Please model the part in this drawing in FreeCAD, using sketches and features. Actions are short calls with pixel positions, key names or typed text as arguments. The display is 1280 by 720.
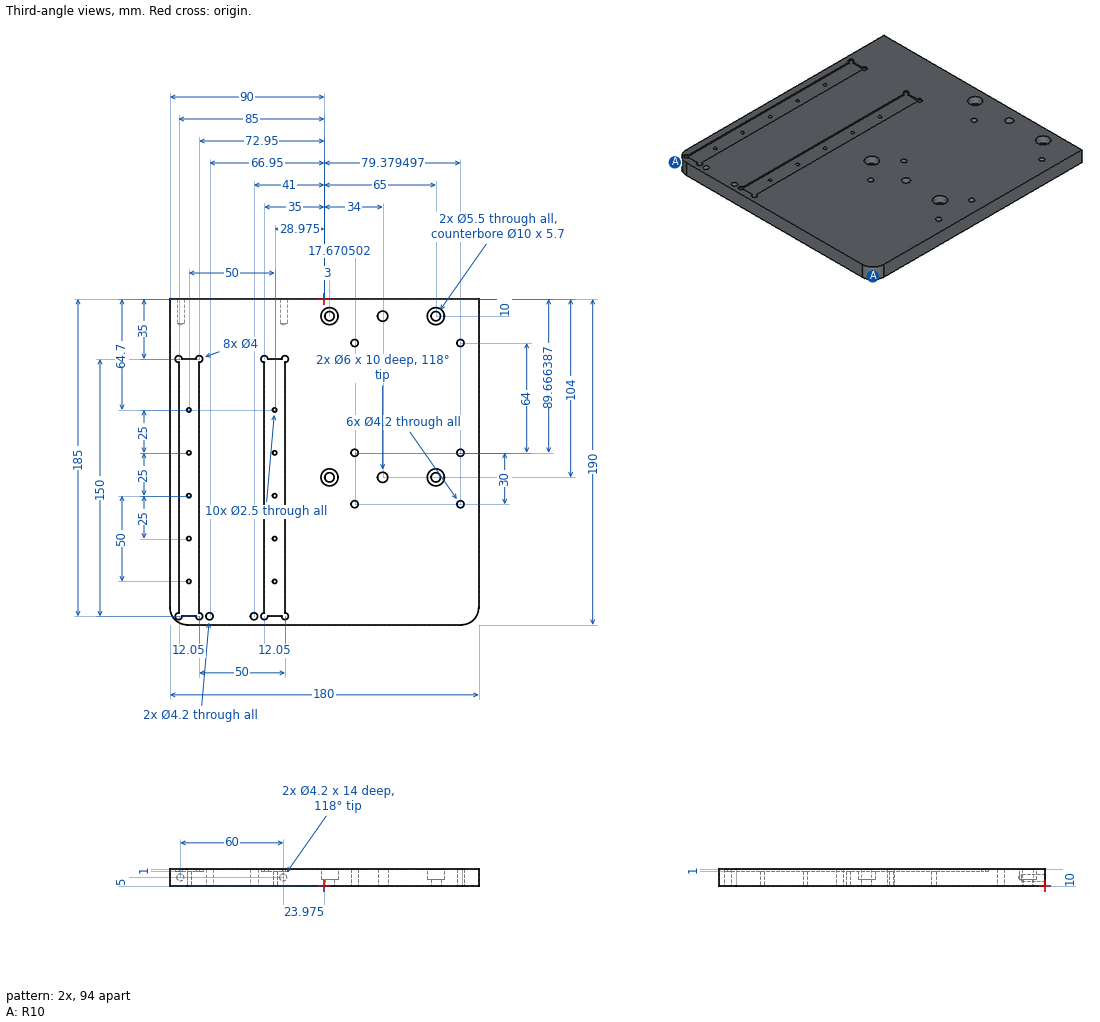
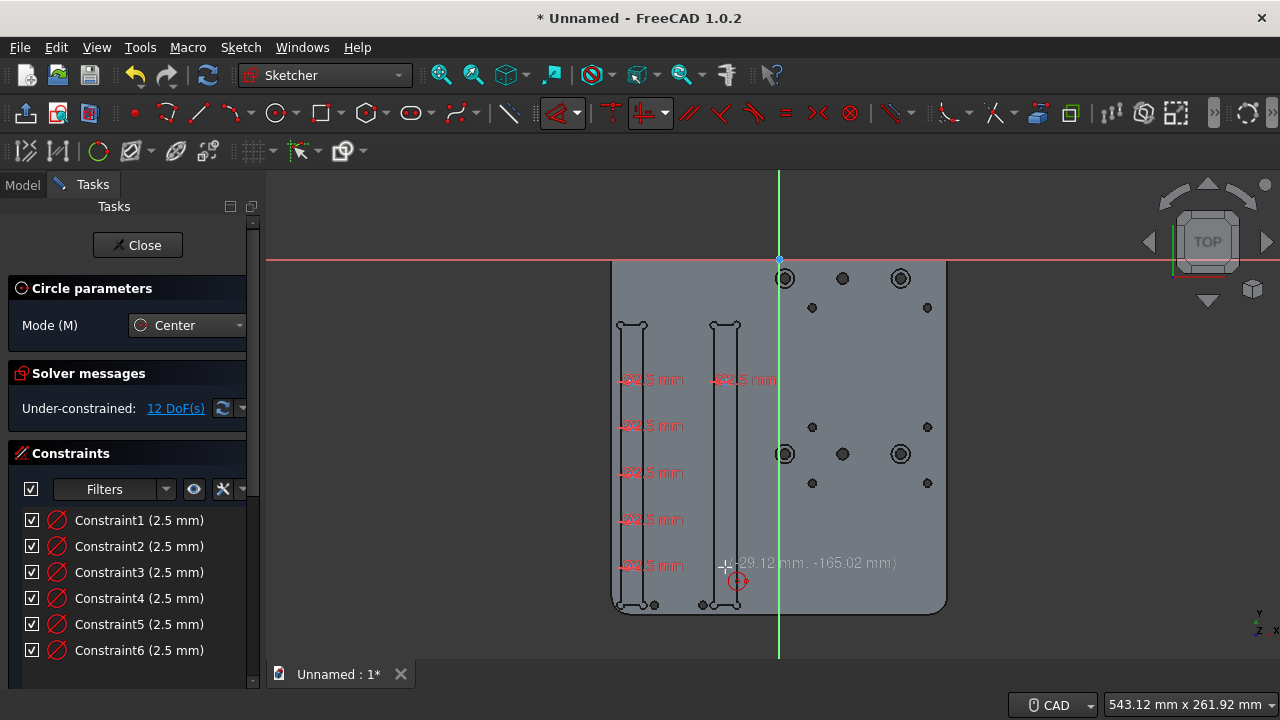
click(725, 567)
move(727, 566)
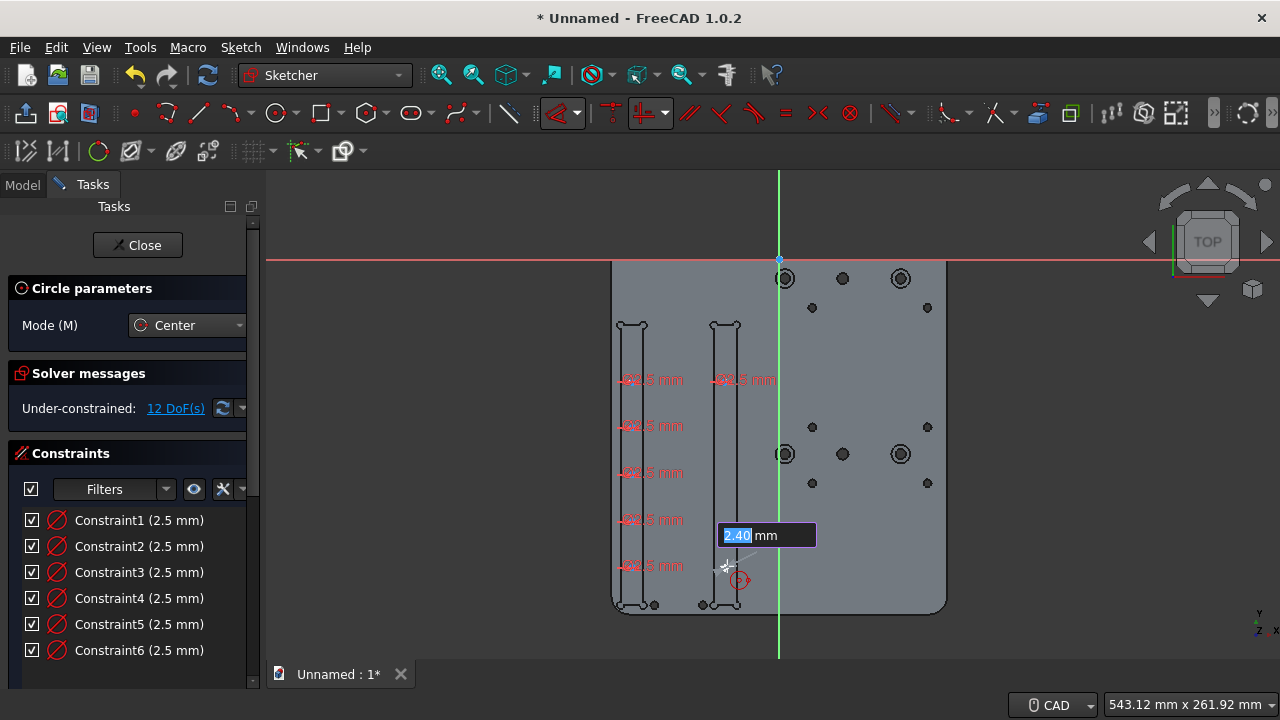
text(2.5)
key(Return)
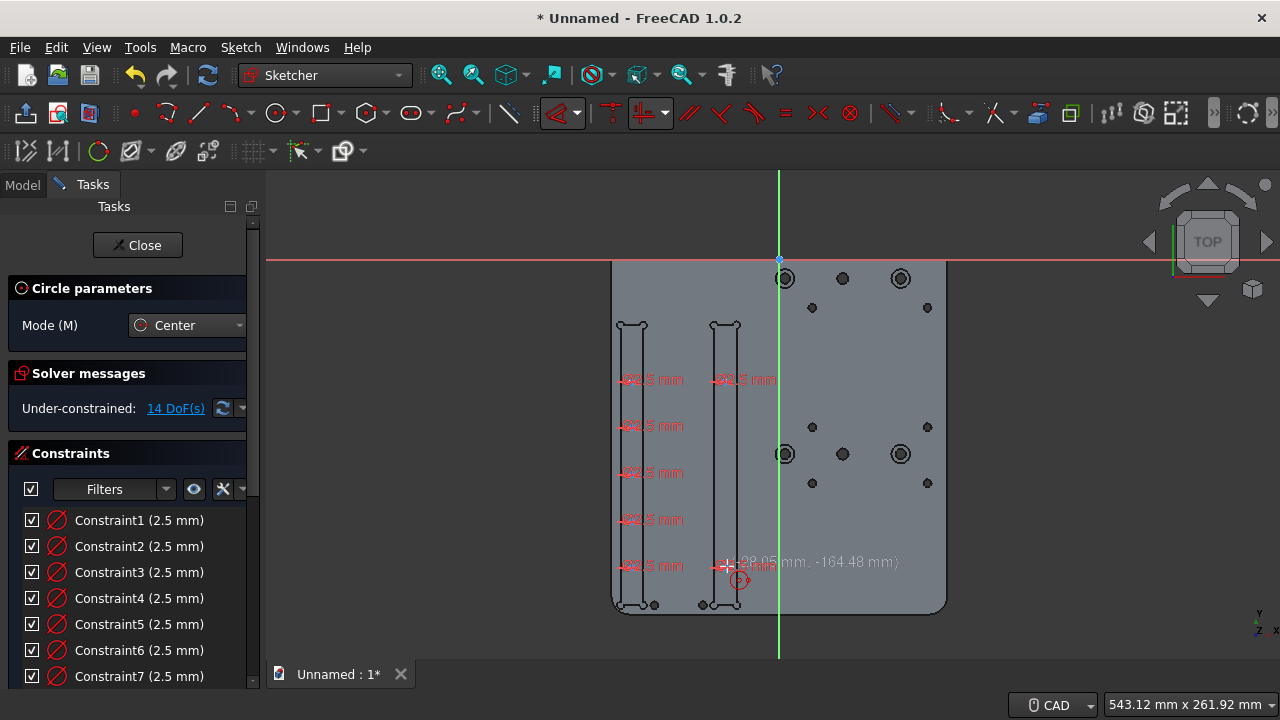
scroll(725, 521, up, 12)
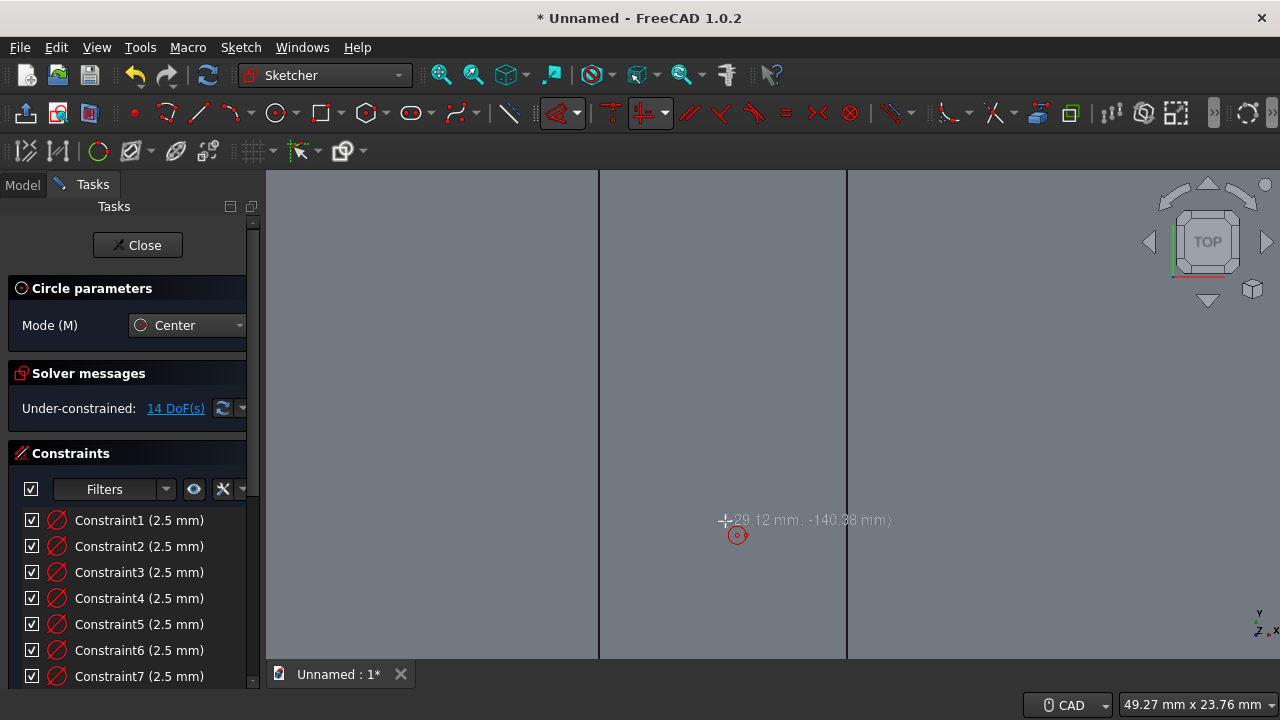
scroll(725, 521, down, 12)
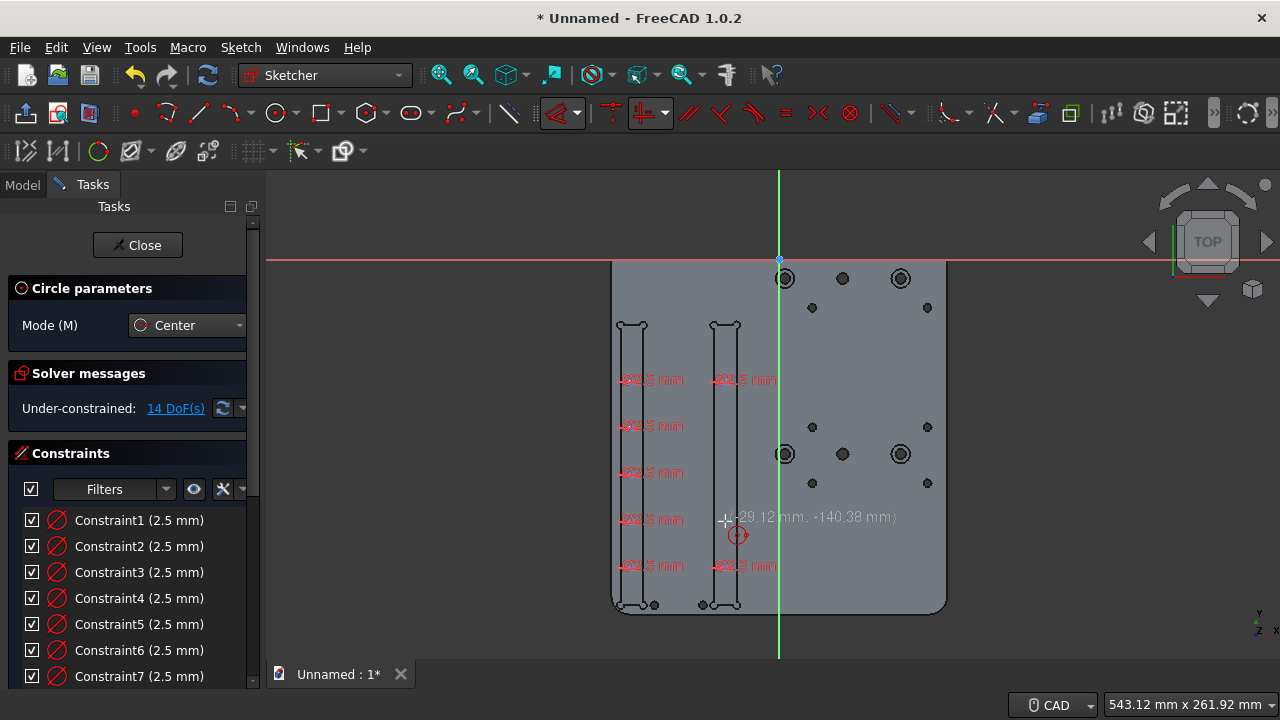
click(725, 521)
move(727, 519)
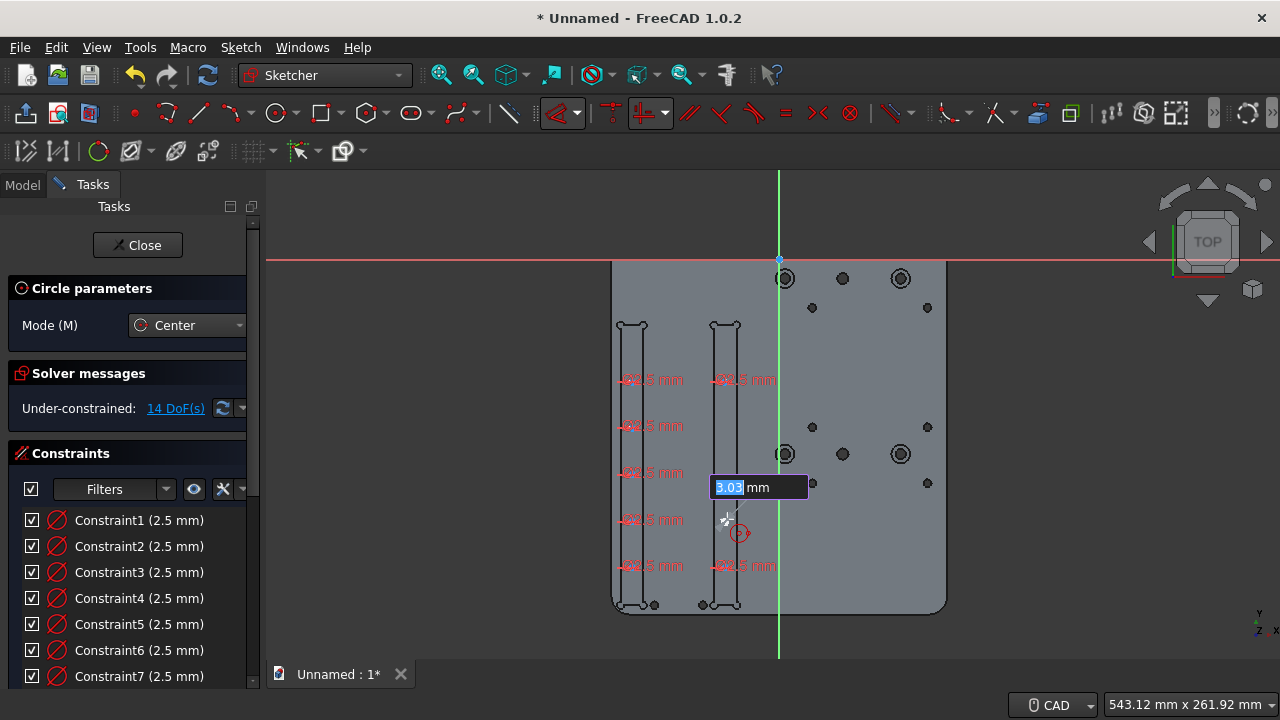
text(2.5)
key(Return)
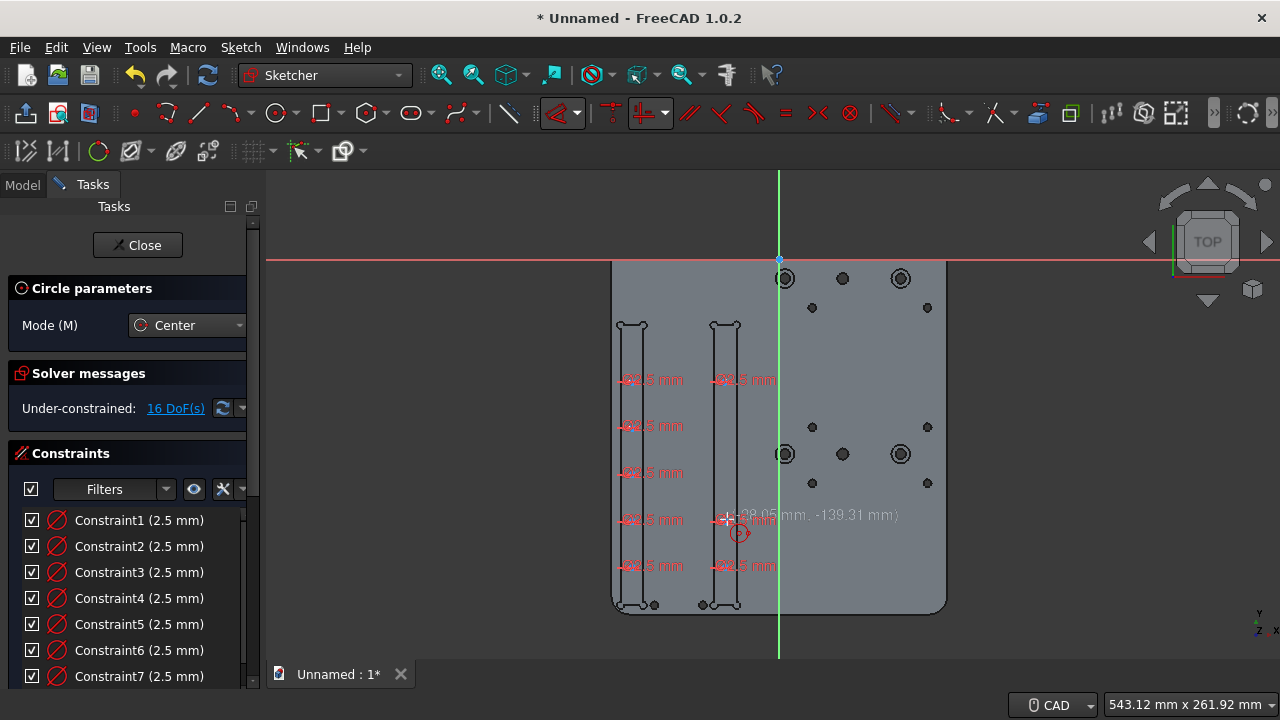
scroll(725, 474, up, 12)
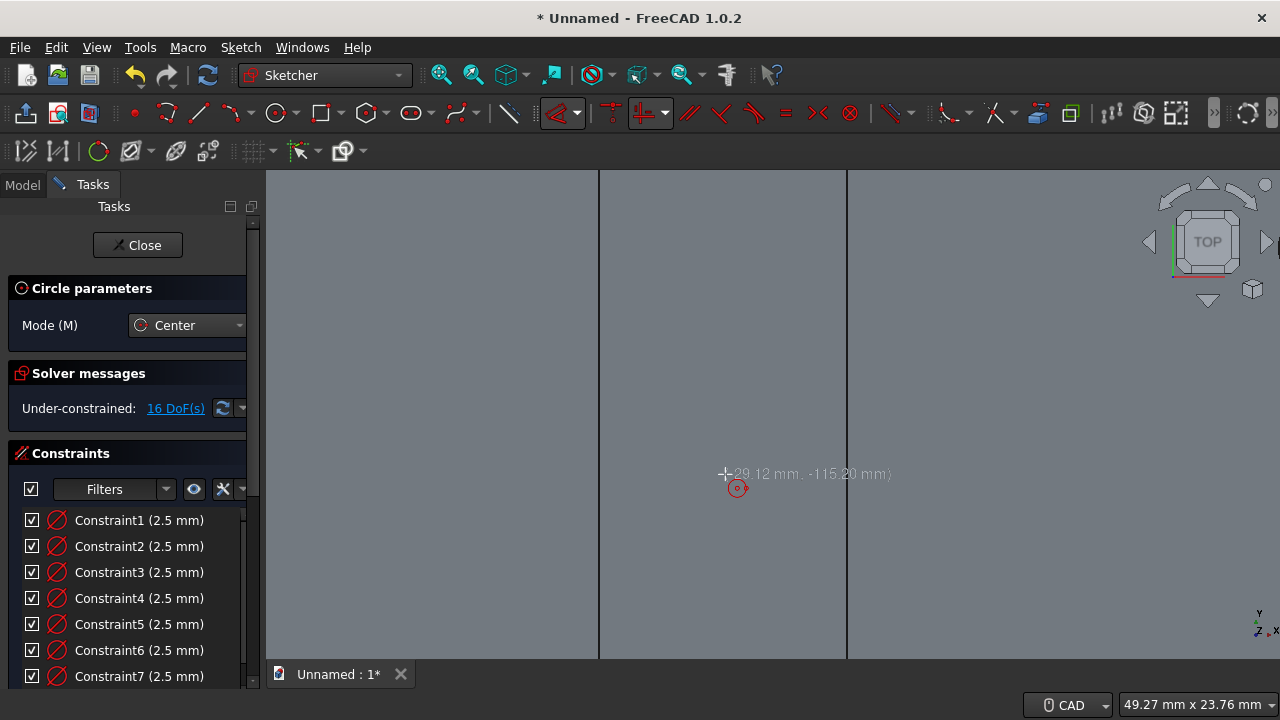
scroll(725, 474, down, 12)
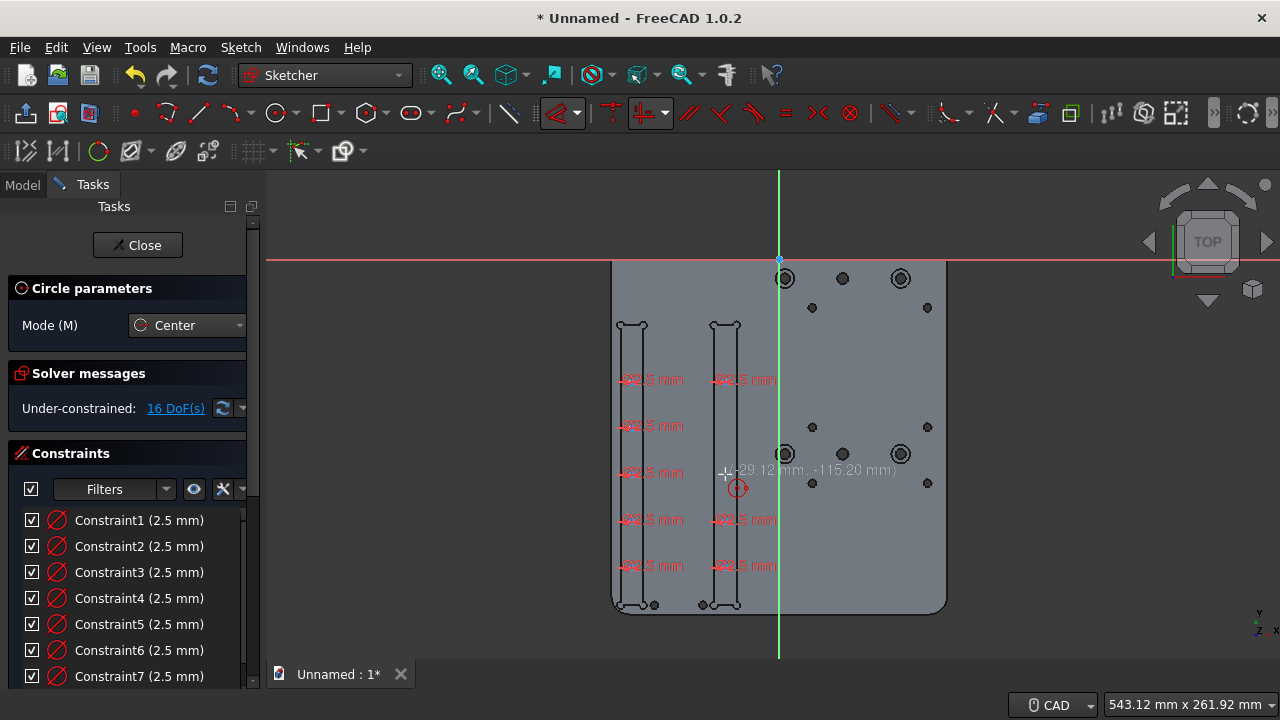
click(725, 474)
move(727, 472)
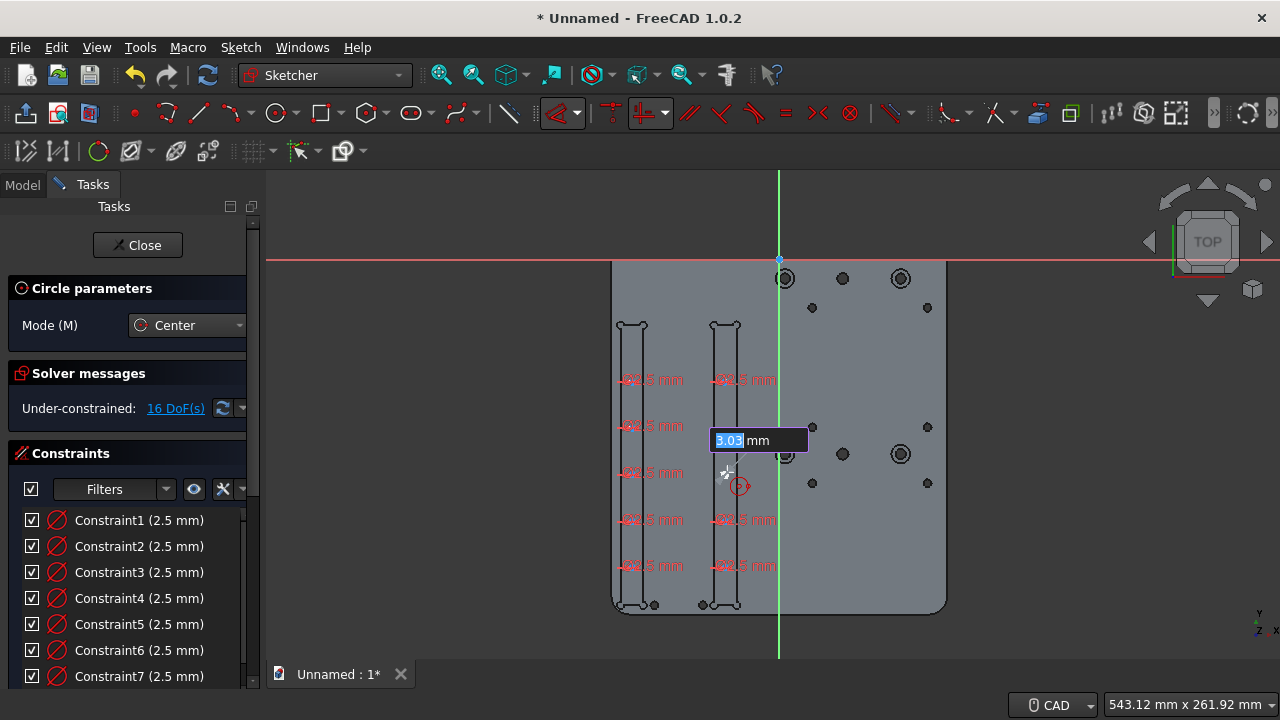
text(2.5)
key(Return)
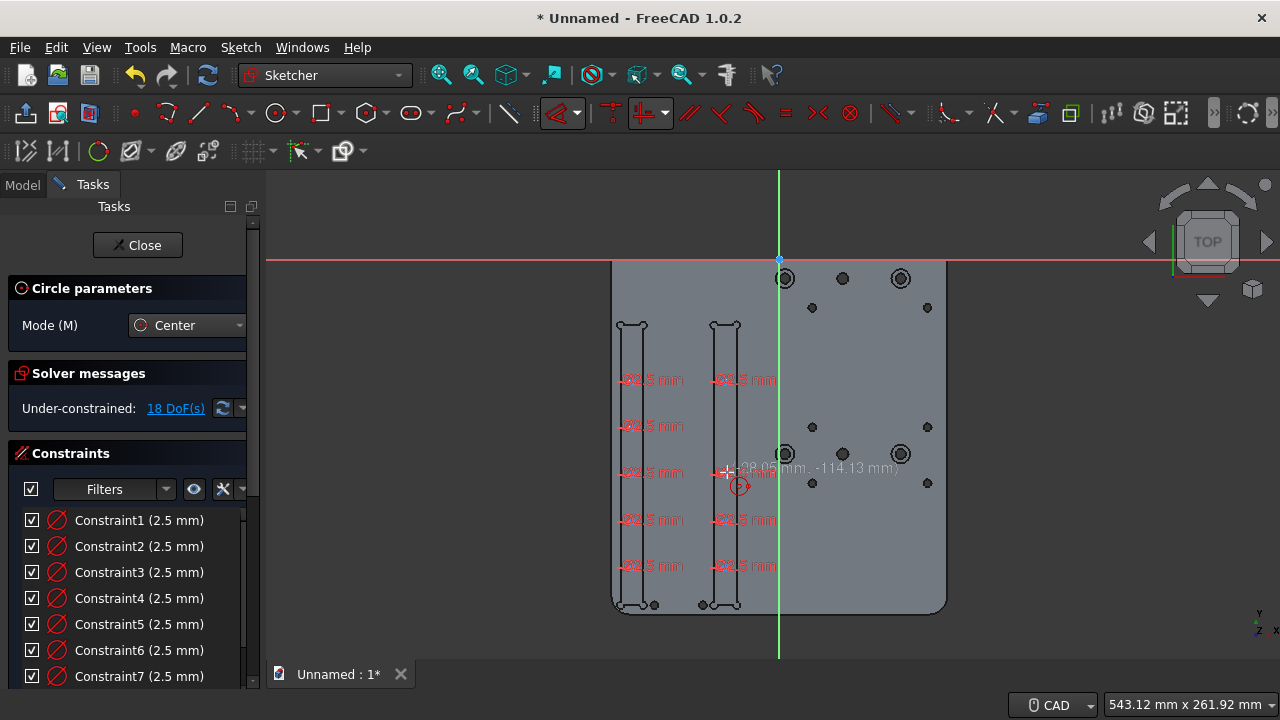
scroll(725, 427, up, 12)